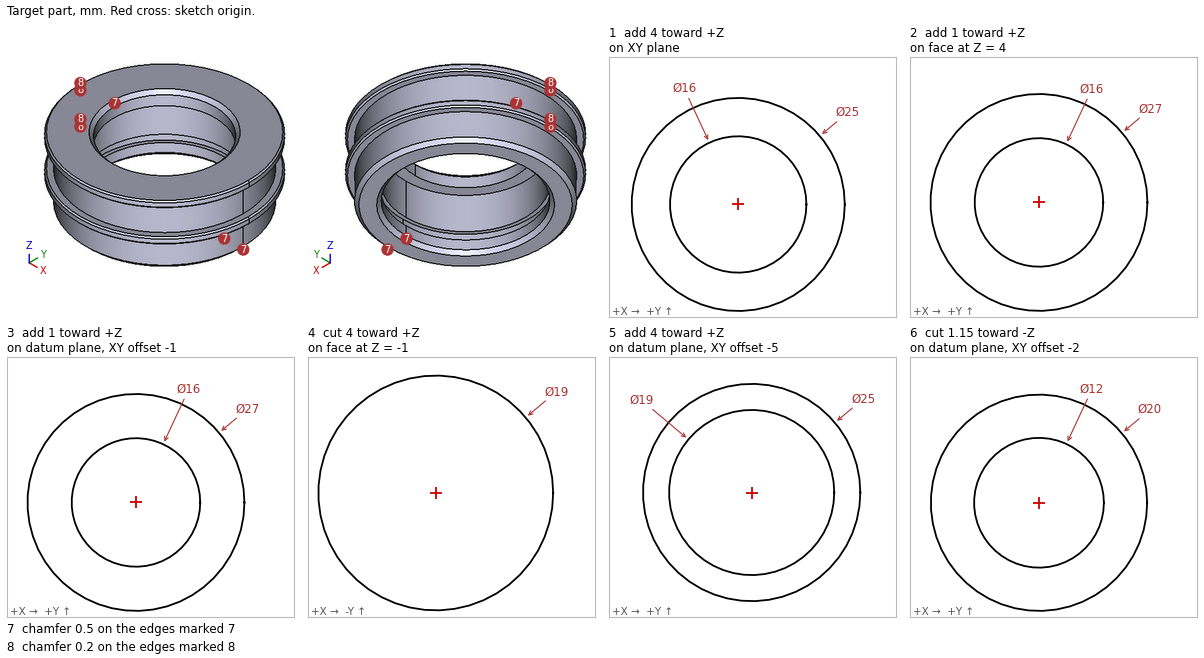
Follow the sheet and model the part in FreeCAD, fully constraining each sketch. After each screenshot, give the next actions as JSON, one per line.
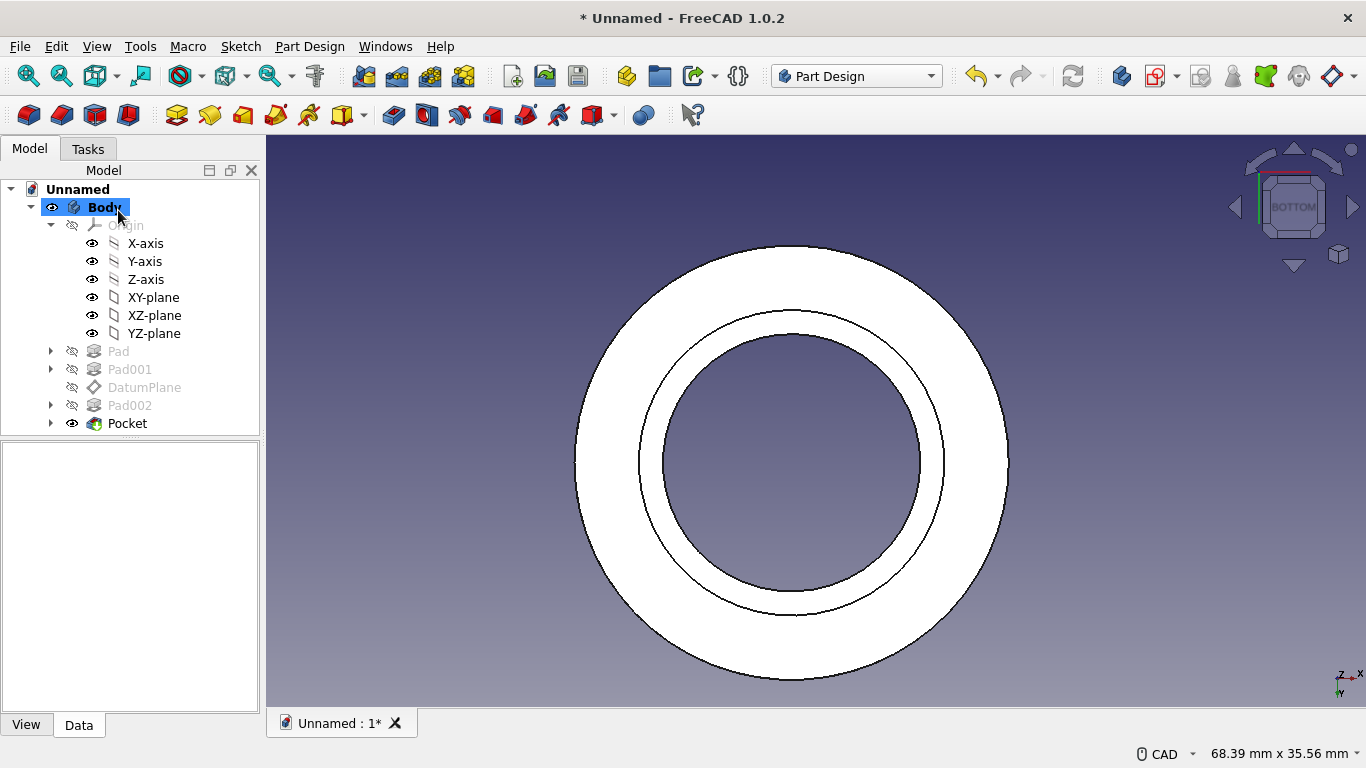
{"action": "left_click", "coordinate": [137, 297]}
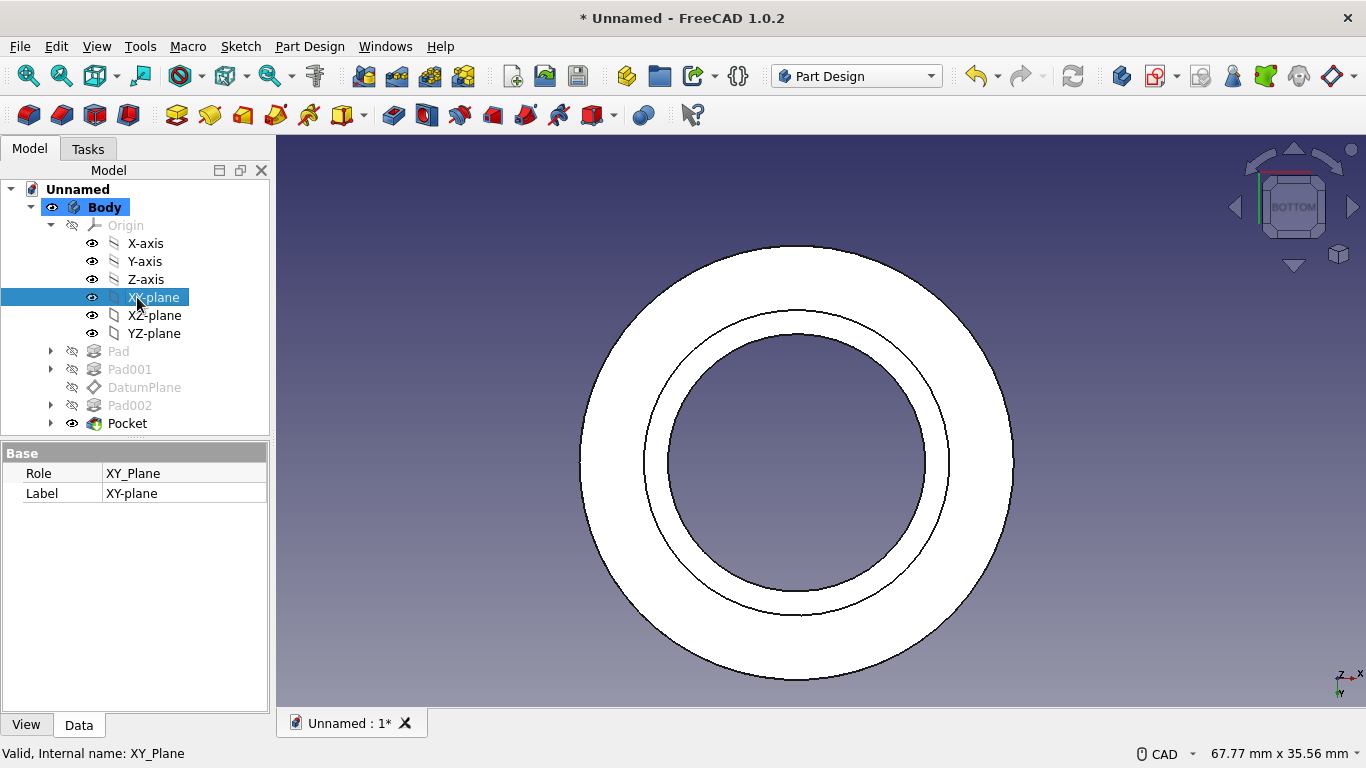
{"action": "left_click", "coordinate": [1332, 76]}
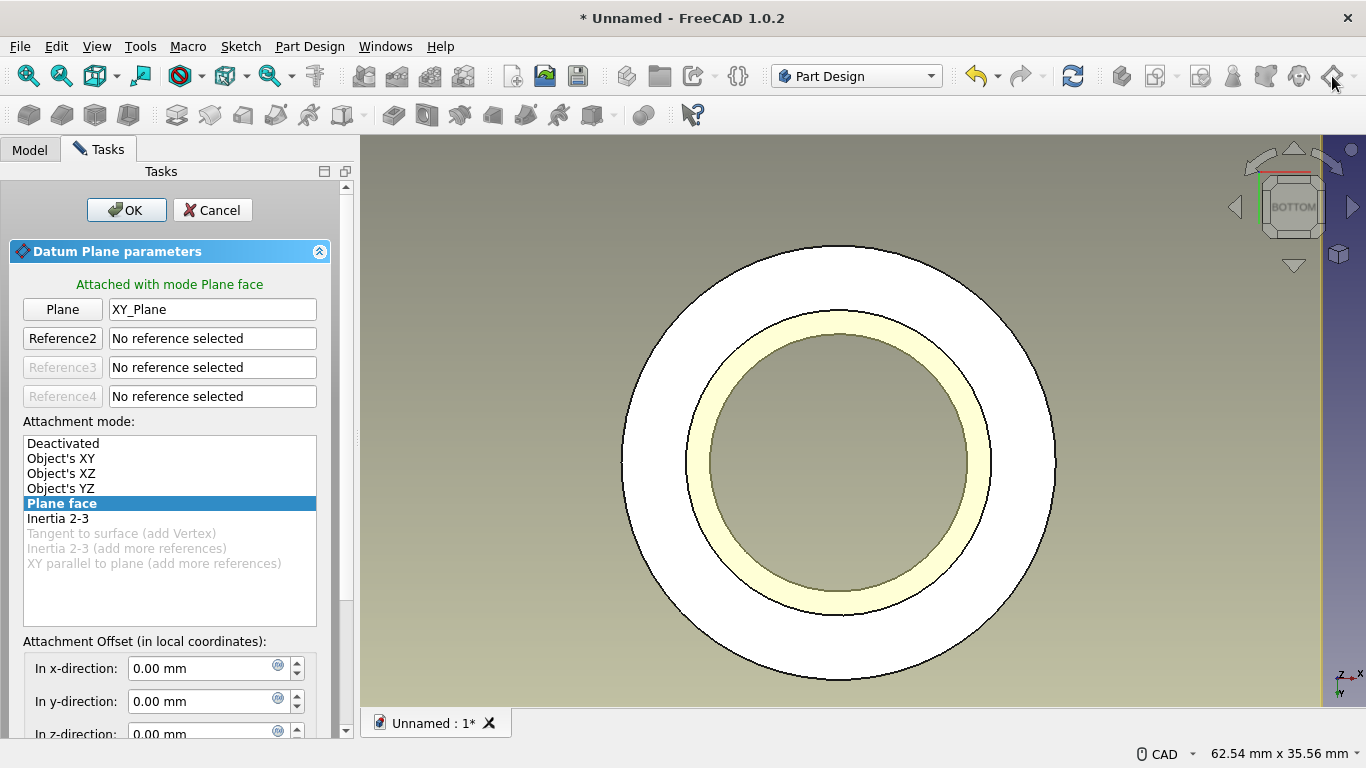
{"action": "scroll", "coordinate": [346, 460], "scroll_direction": "down", "scroll_amount": 2}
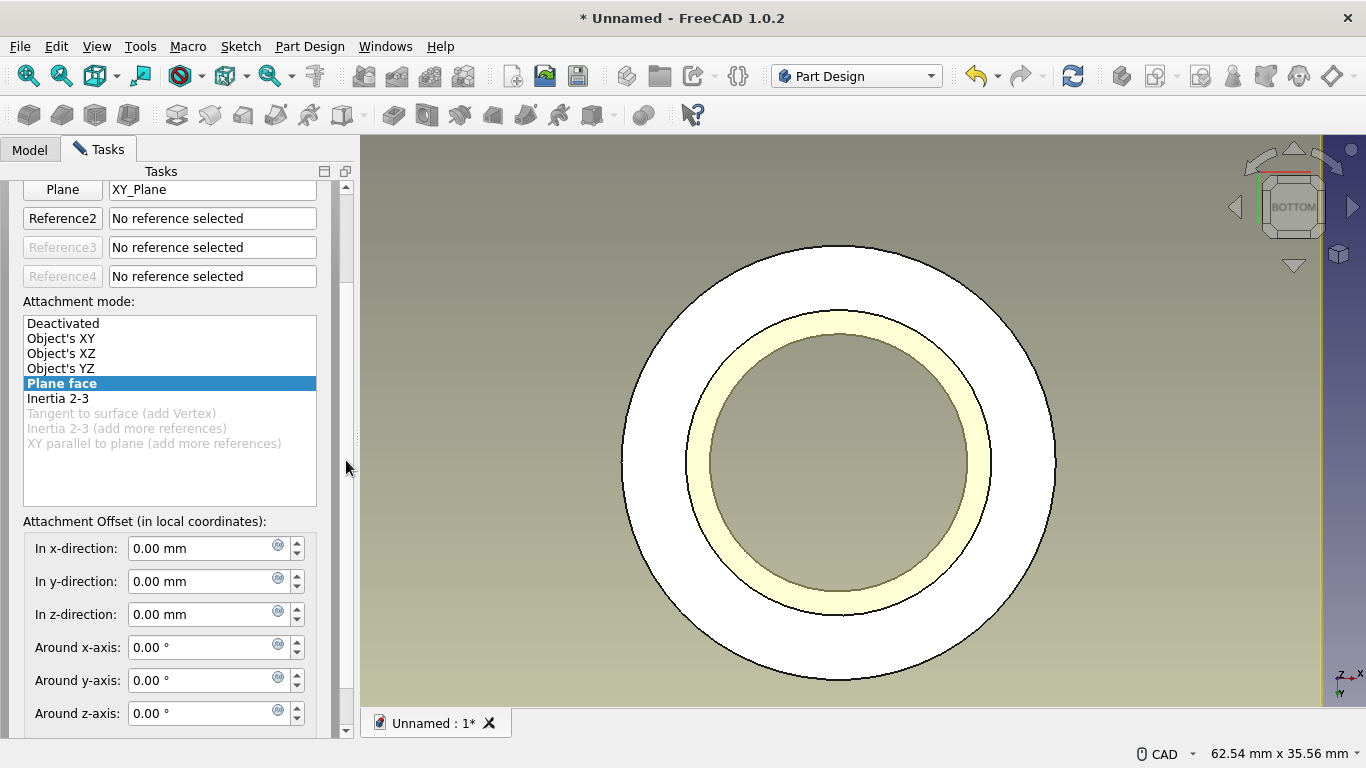
{"action": "triple_click", "coordinate": [210, 614]}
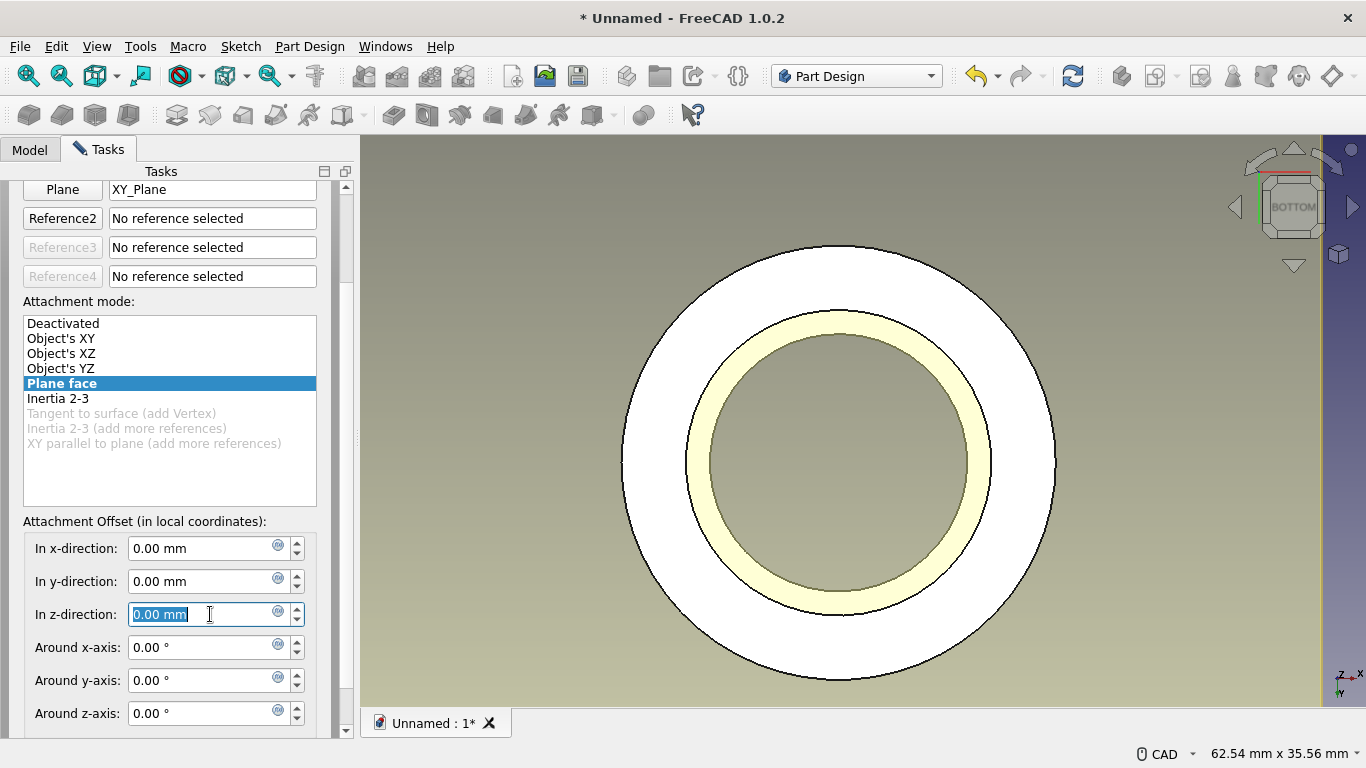
{"action": "type", "text": "-5"}
{"action": "key", "text": "Tab"}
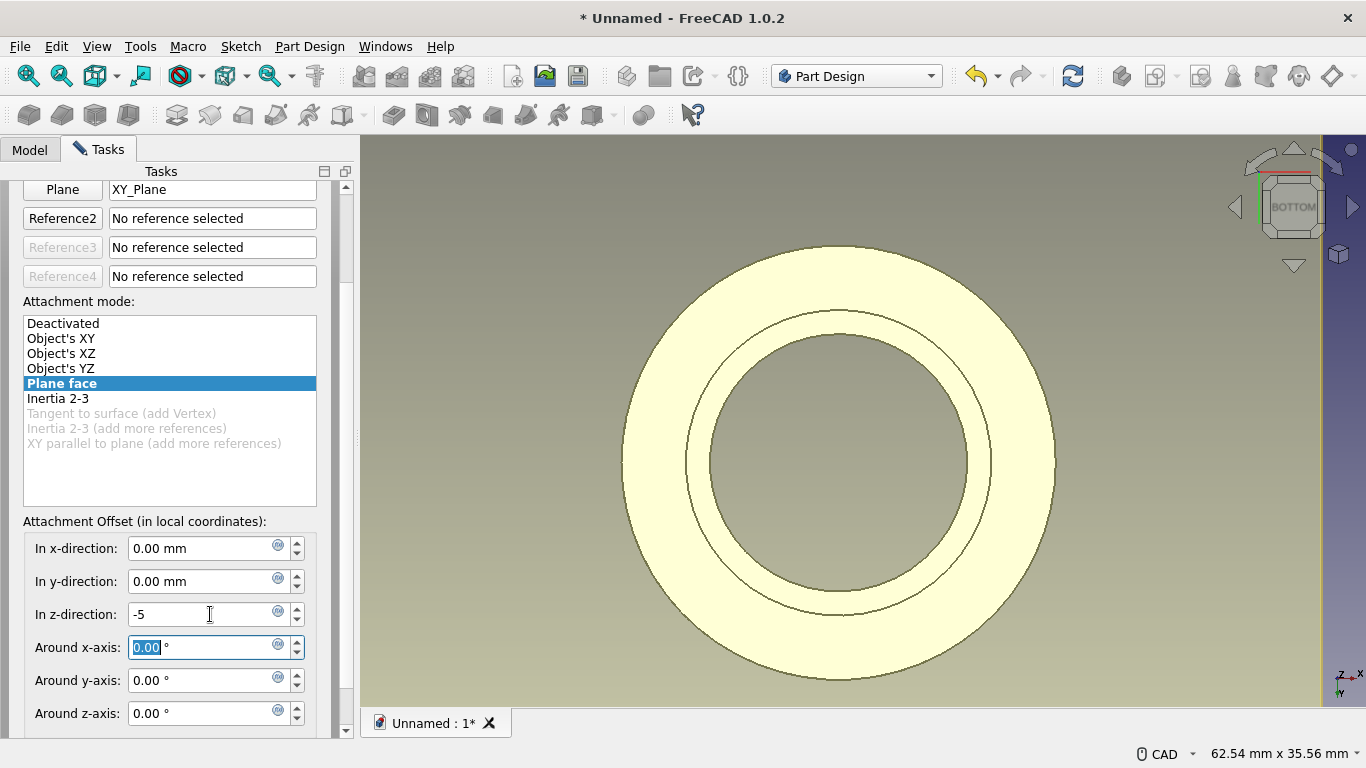
{"action": "scroll", "coordinate": [346, 460], "scroll_direction": "up", "scroll_amount": 3}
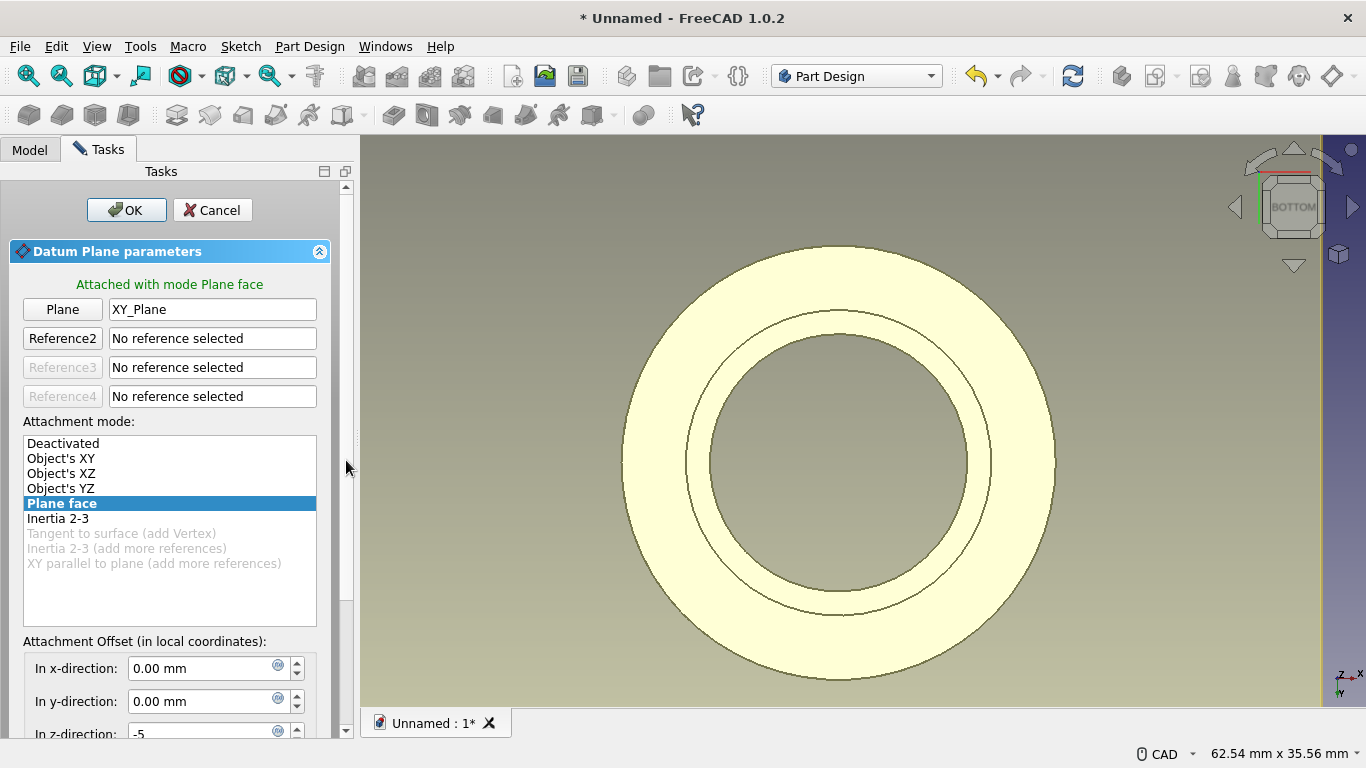
{"action": "left_click", "coordinate": [127, 210]}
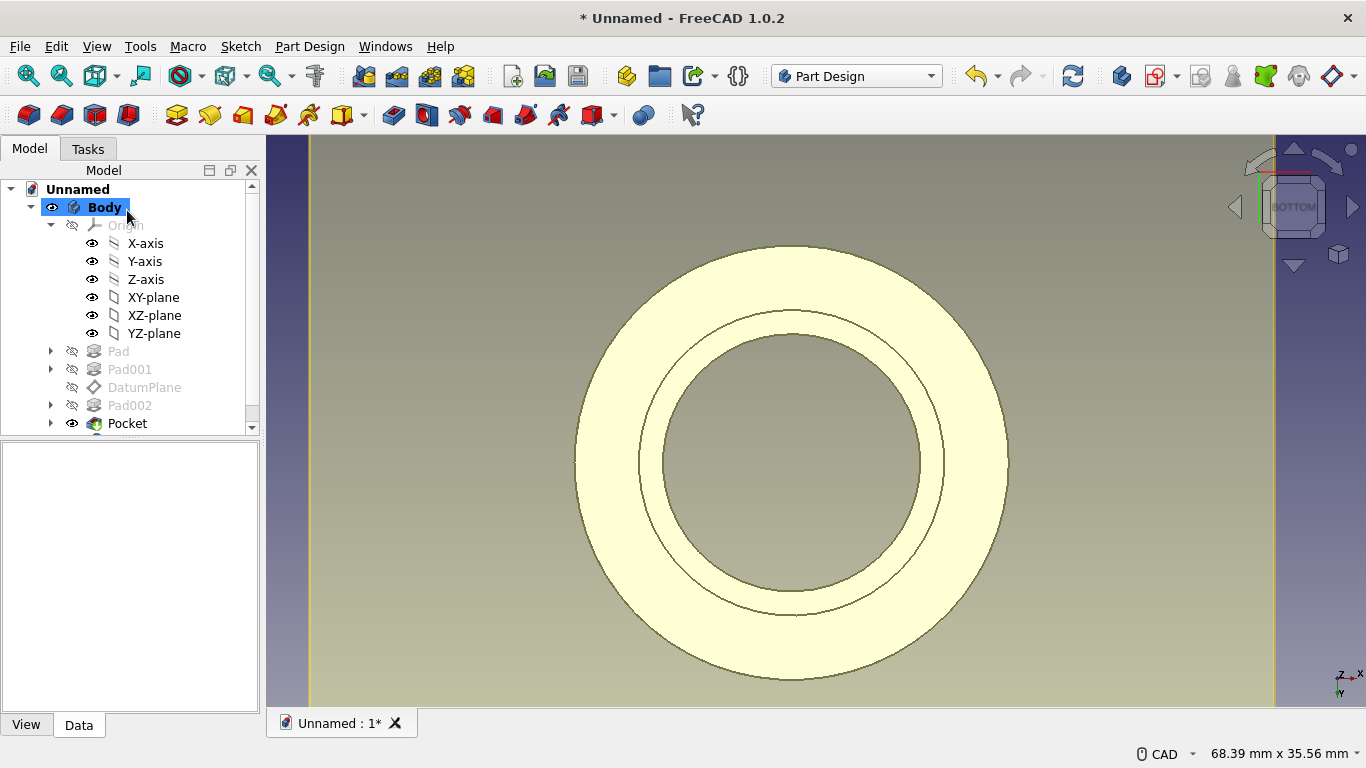
{"action": "scroll", "coordinate": [101, 311], "scroll_direction": "down", "scroll_amount": 3}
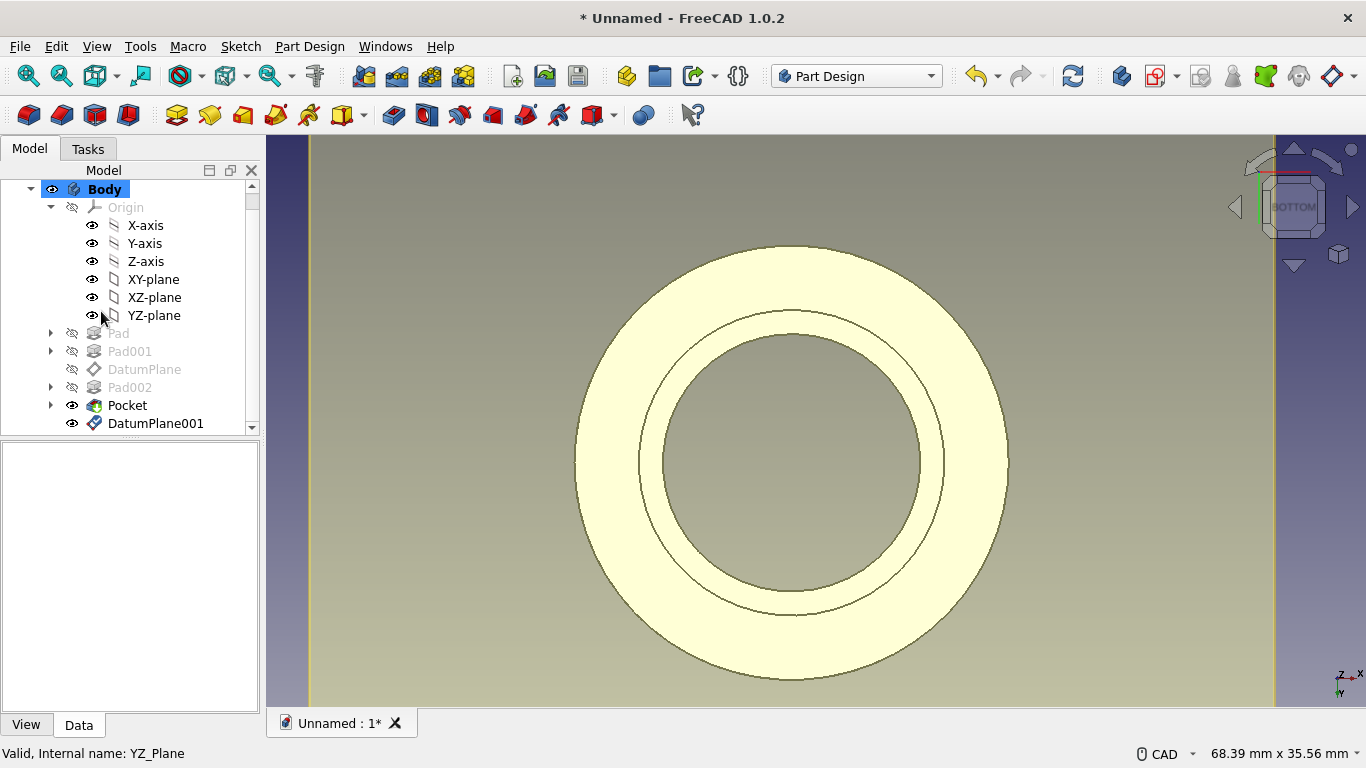
{"action": "left_click", "coordinate": [117, 423]}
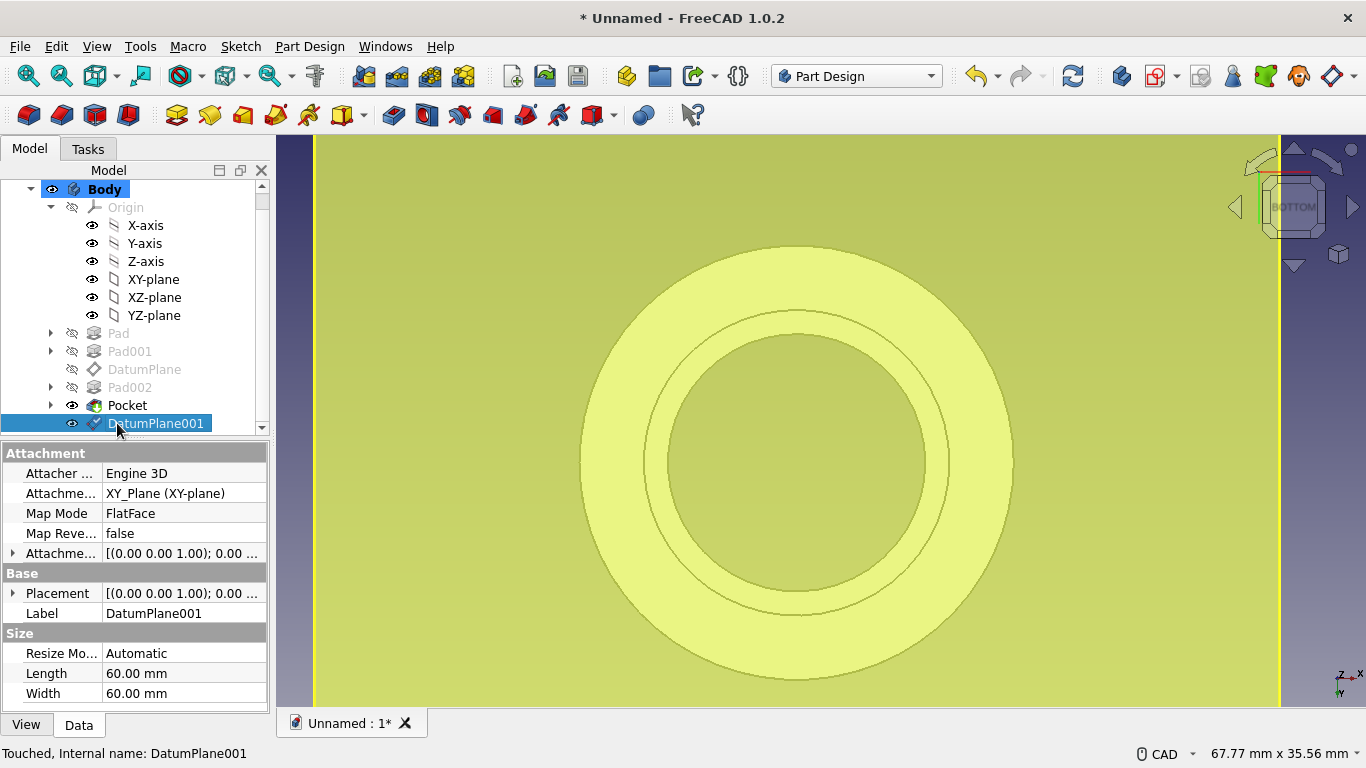
{"action": "left_click", "coordinate": [1154, 76]}